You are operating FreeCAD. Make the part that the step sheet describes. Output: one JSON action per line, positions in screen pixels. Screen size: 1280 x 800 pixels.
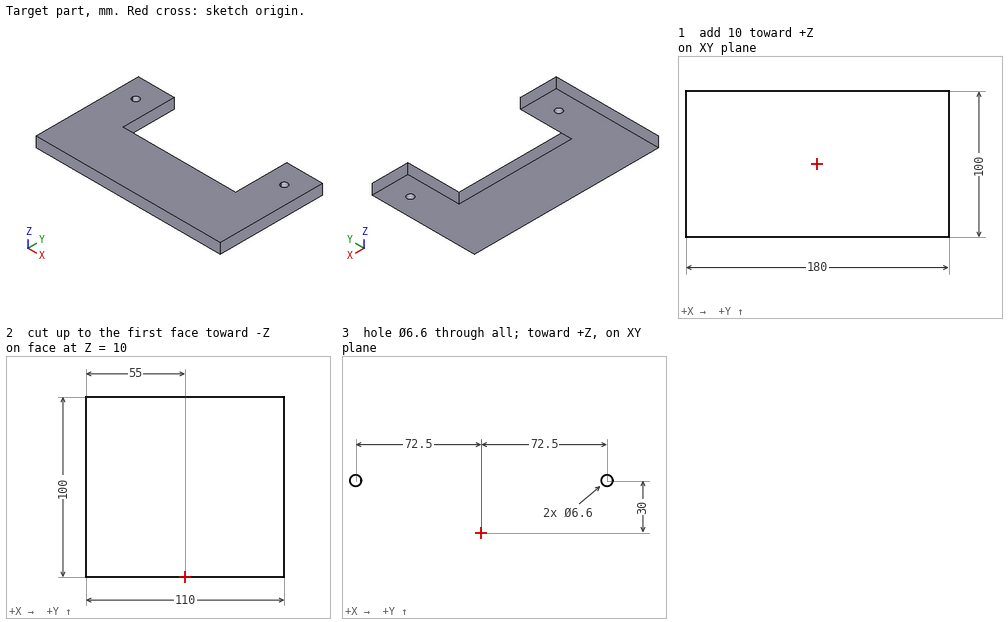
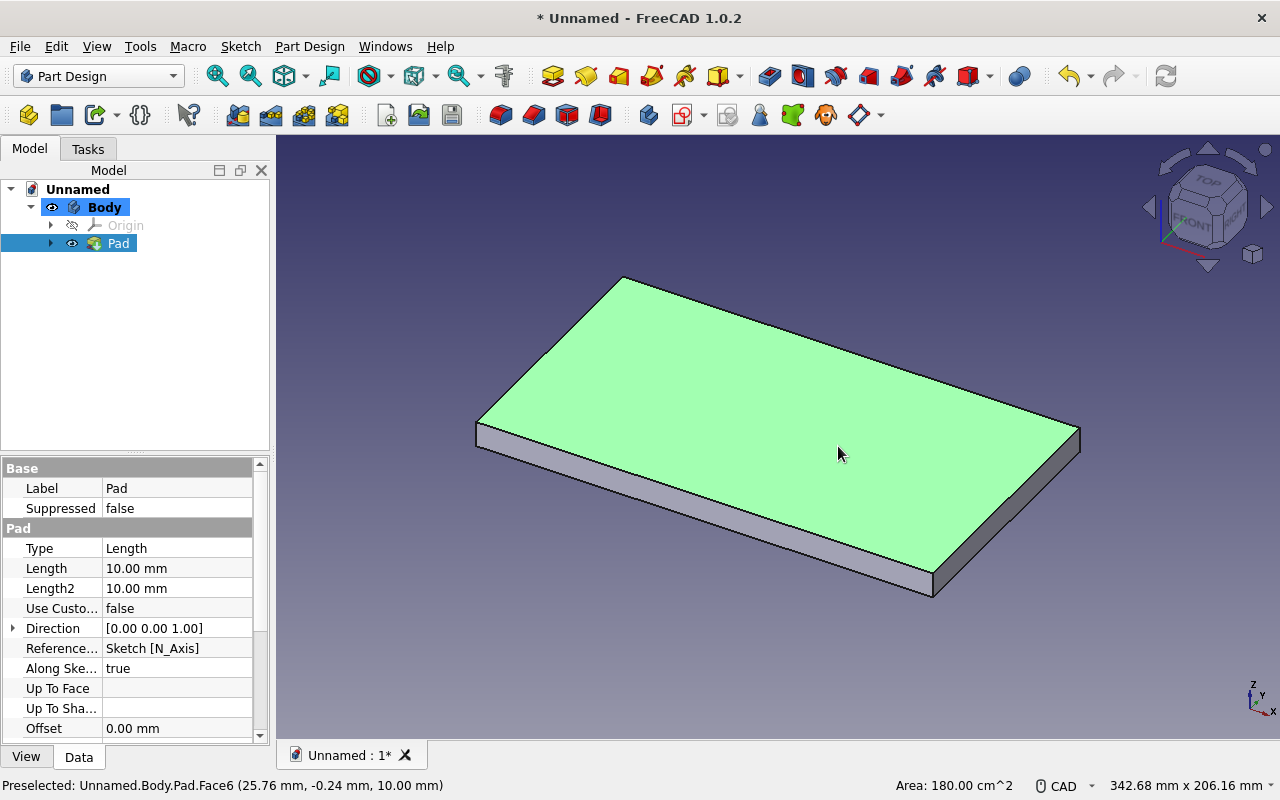
{"action": "left_click", "coordinate": [682, 116]}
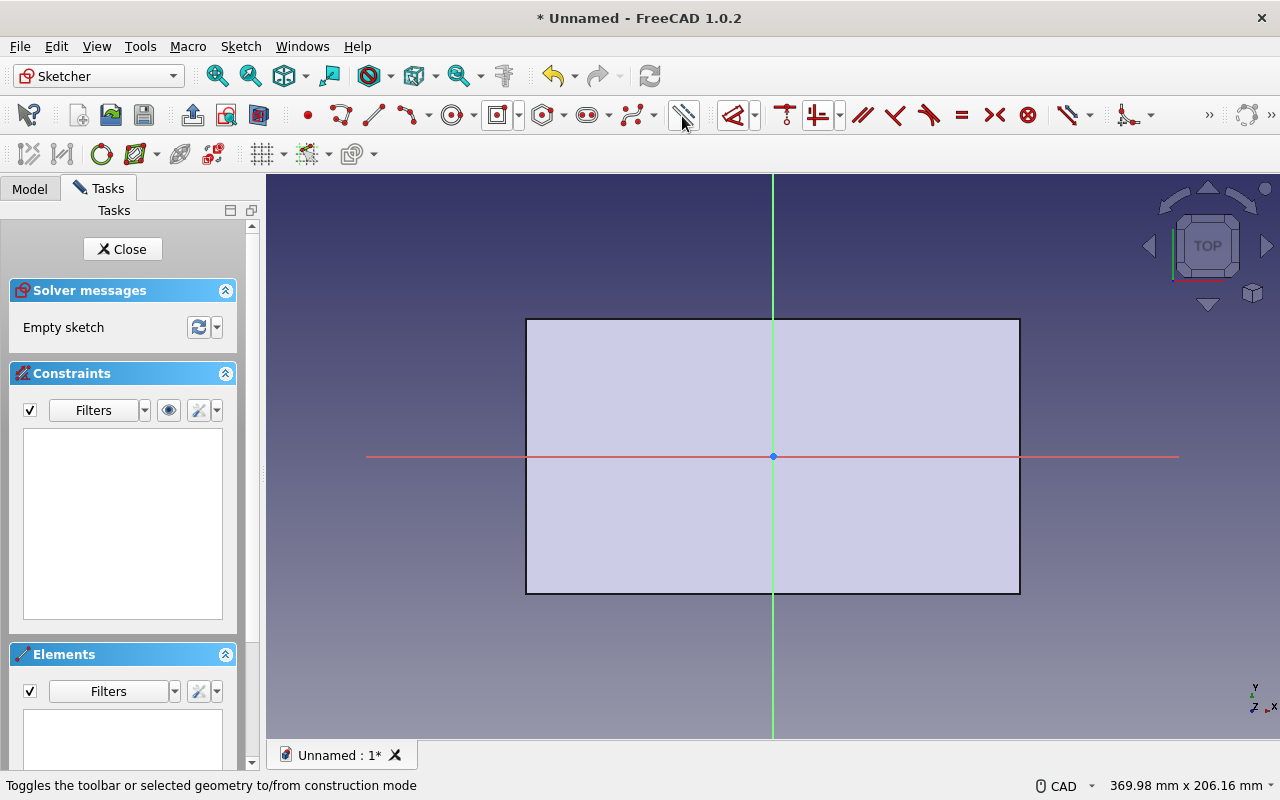
{"action": "scroll", "coordinate": [395, 711], "scroll_direction": "down", "scroll_amount": 1}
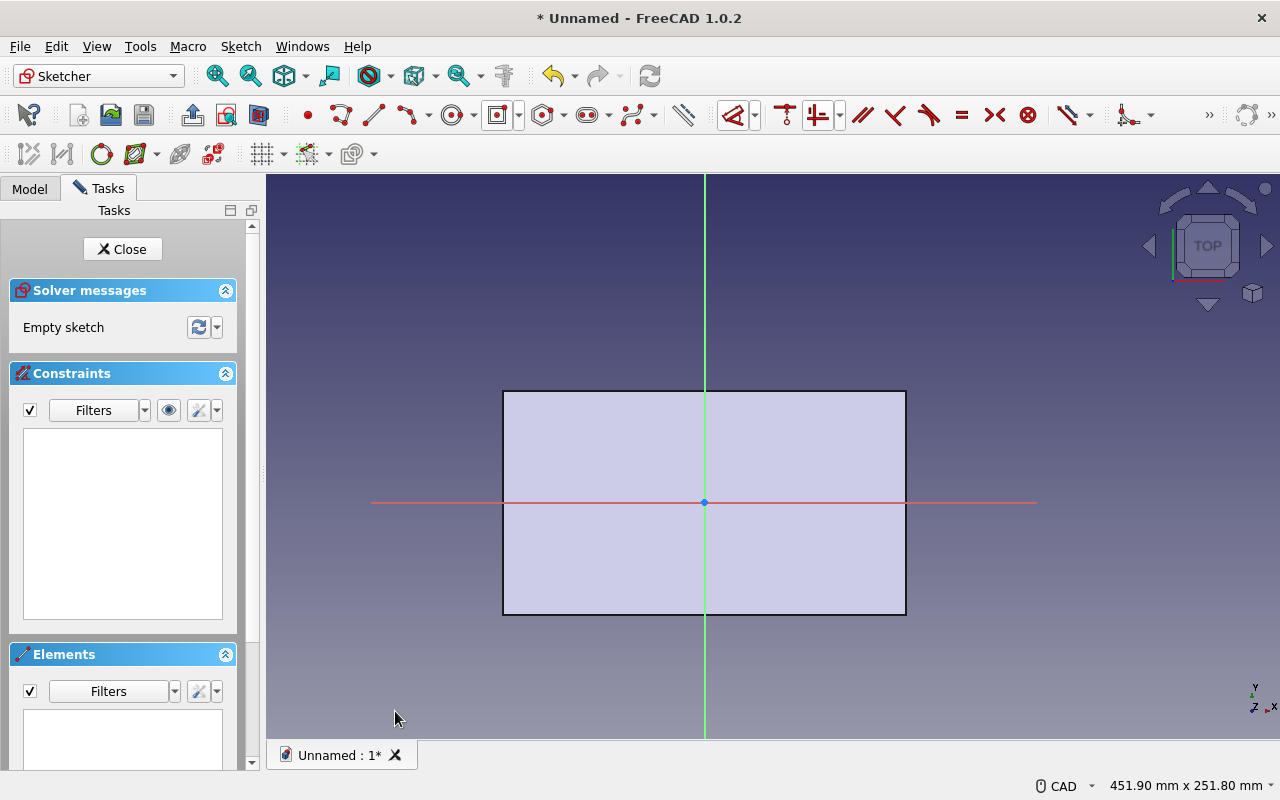
{"action": "scroll", "coordinate": [705, 257], "scroll_direction": "up", "scroll_amount": 2}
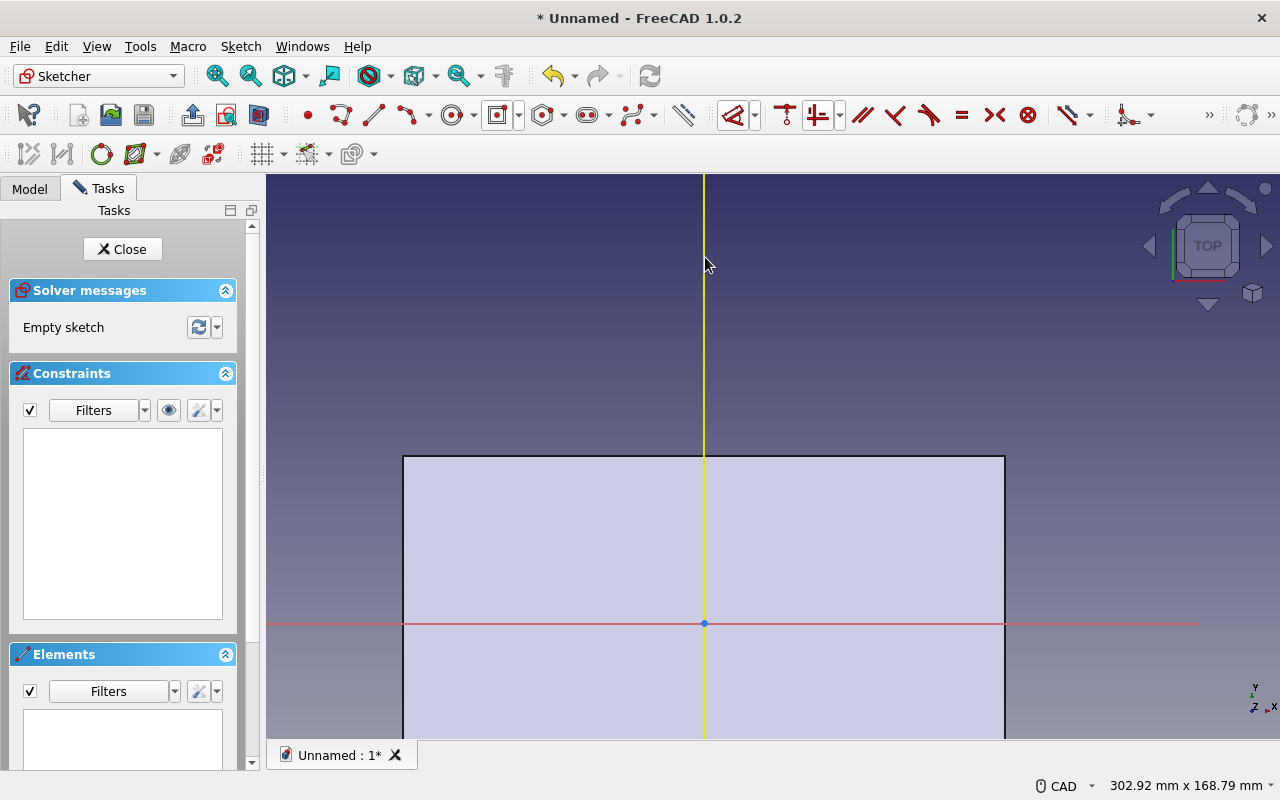
{"action": "key", "text": "g r"}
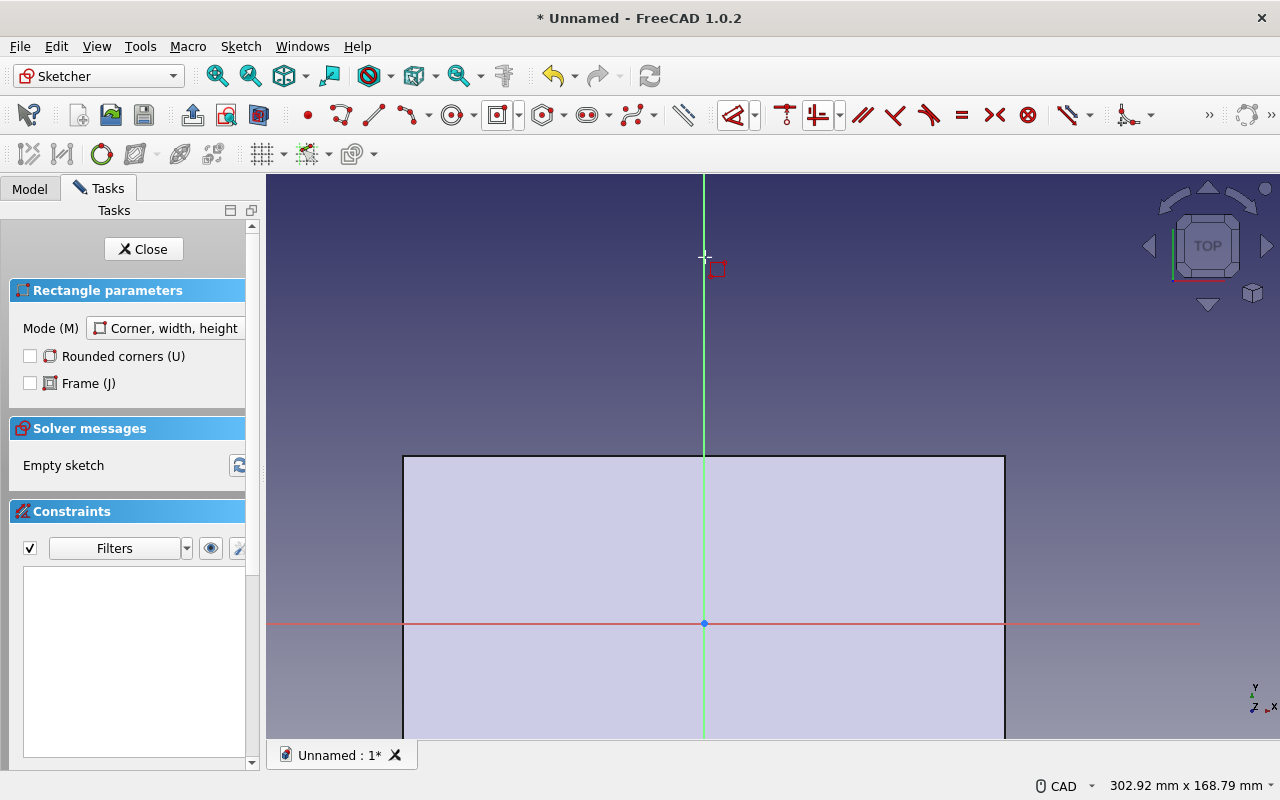
{"action": "left_click", "coordinate": [520, 289]}
{"action": "left_click", "coordinate": [888, 624]}
{"action": "key", "text": "Escape"}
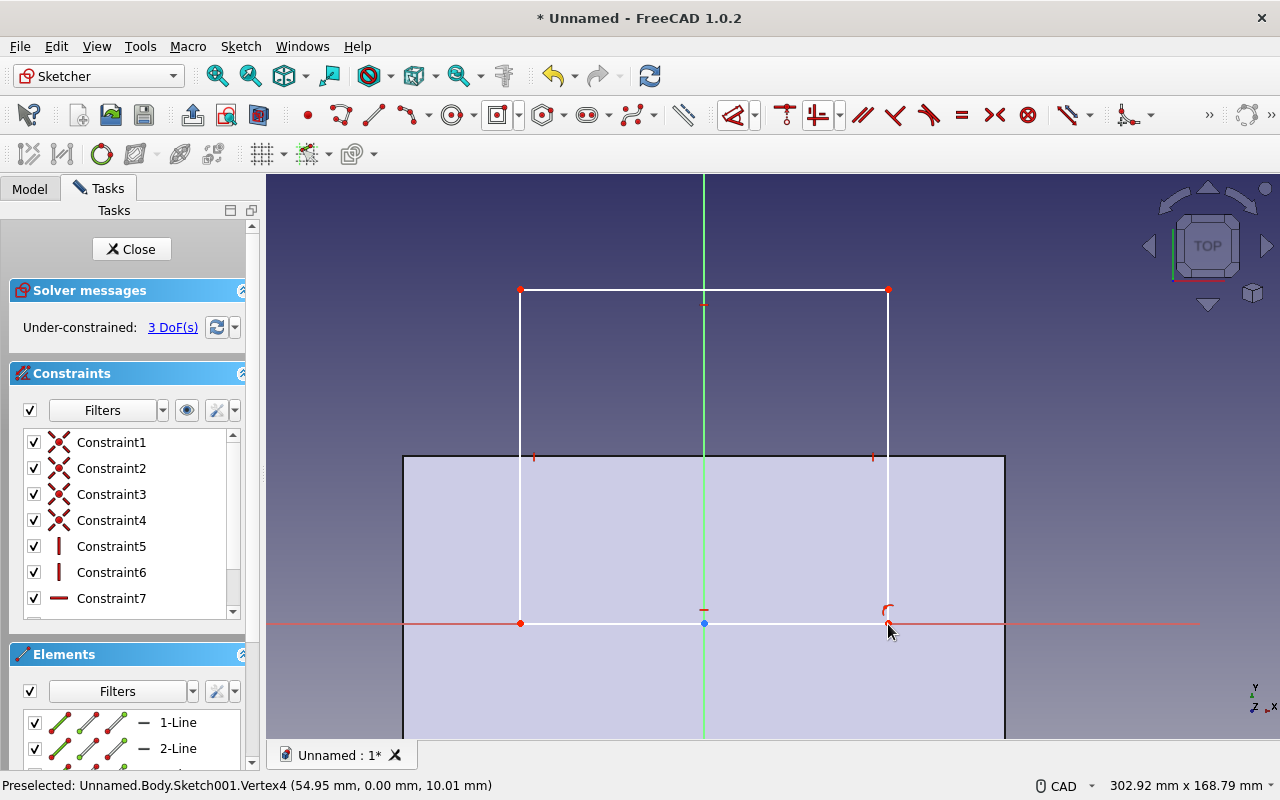
{"action": "left_click", "coordinate": [520, 390]}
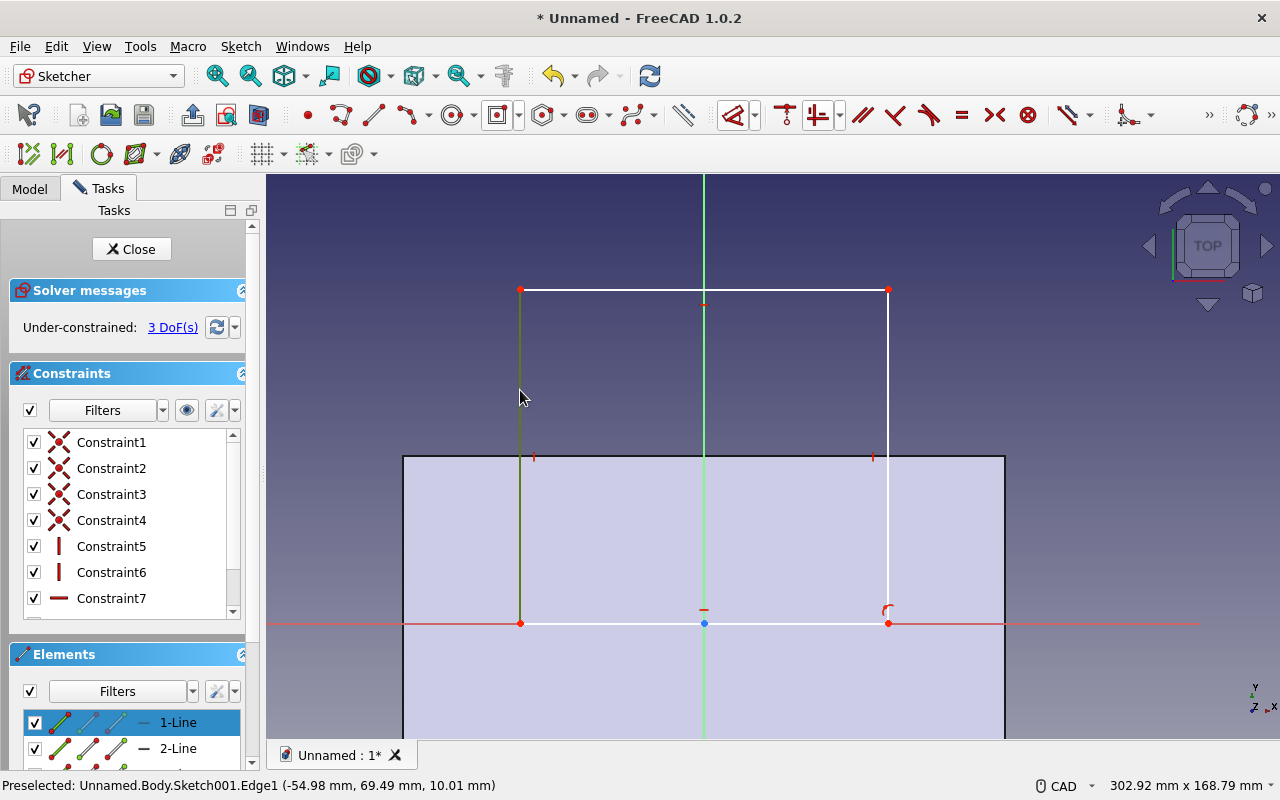
{"action": "key", "text": "i"}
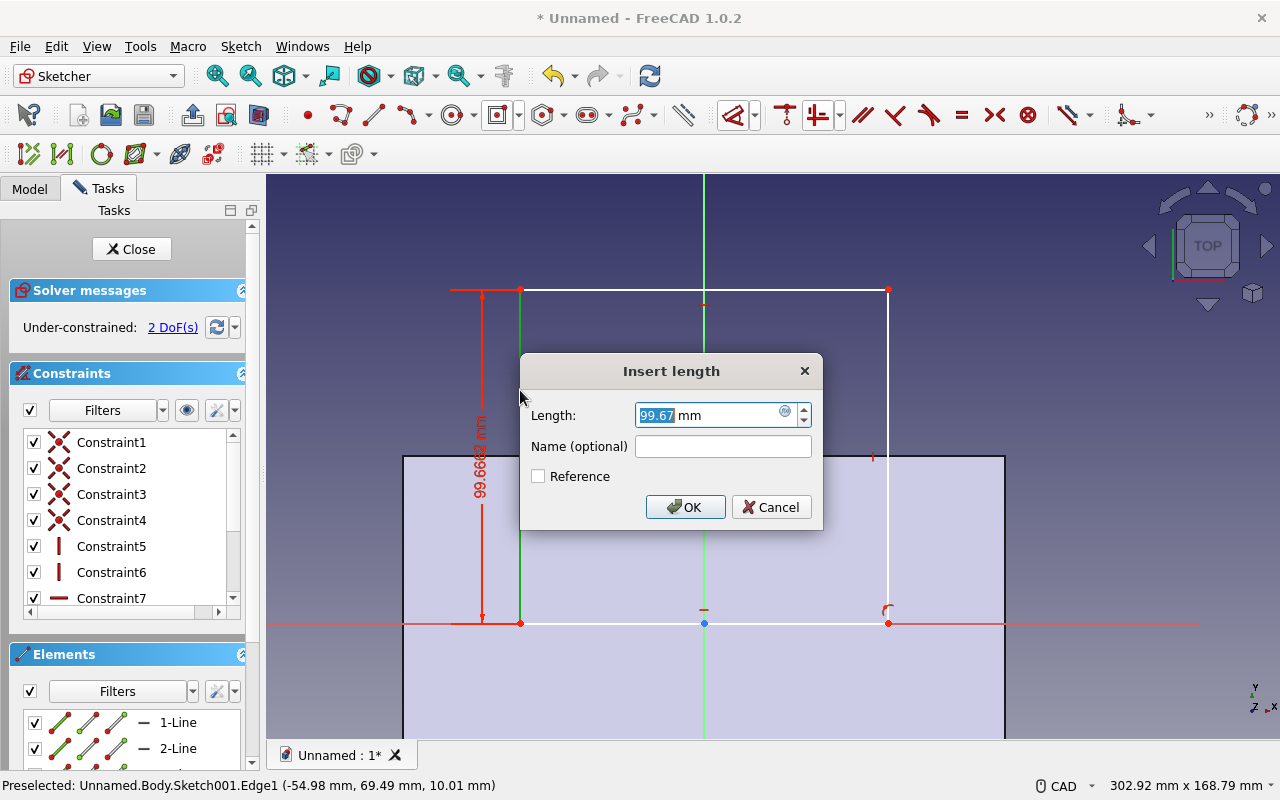
{"action": "type", "text": "100"}
{"action": "key", "text": "Return"}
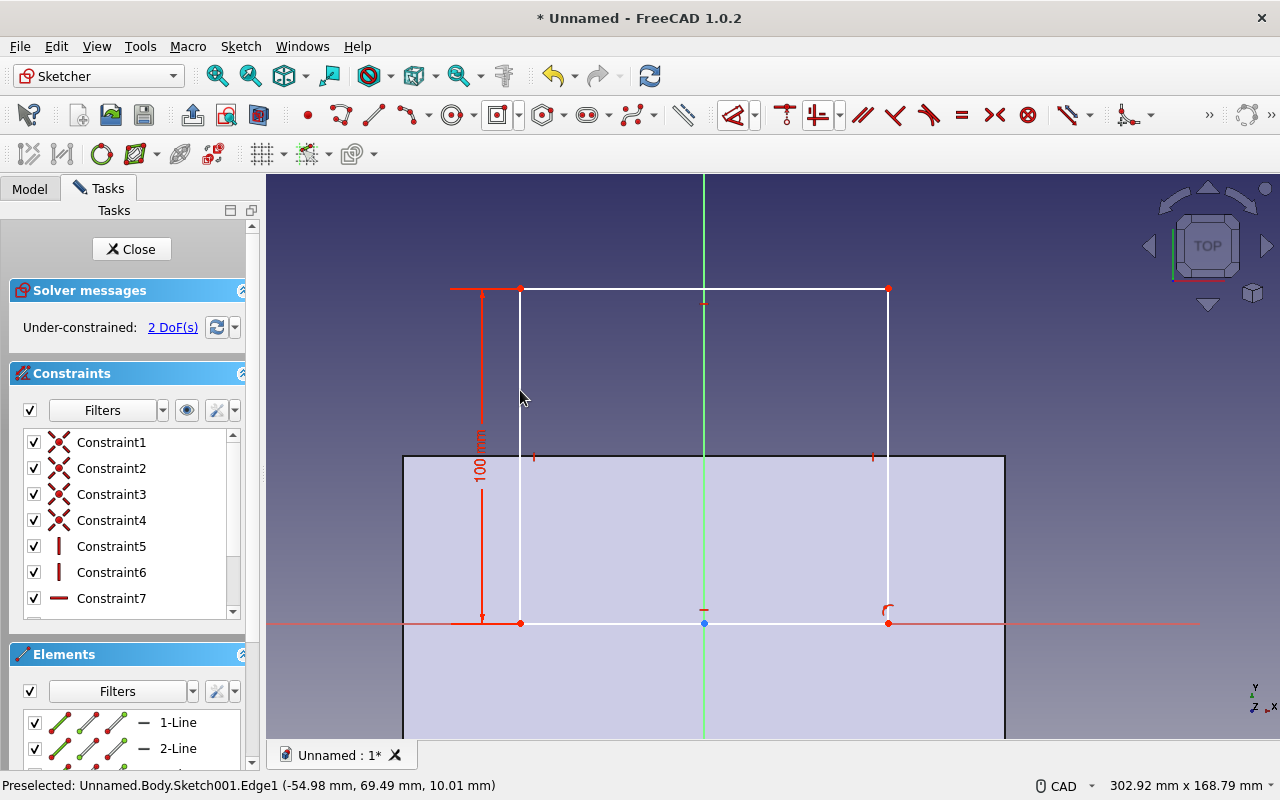
{"action": "left_click", "coordinate": [630, 624]}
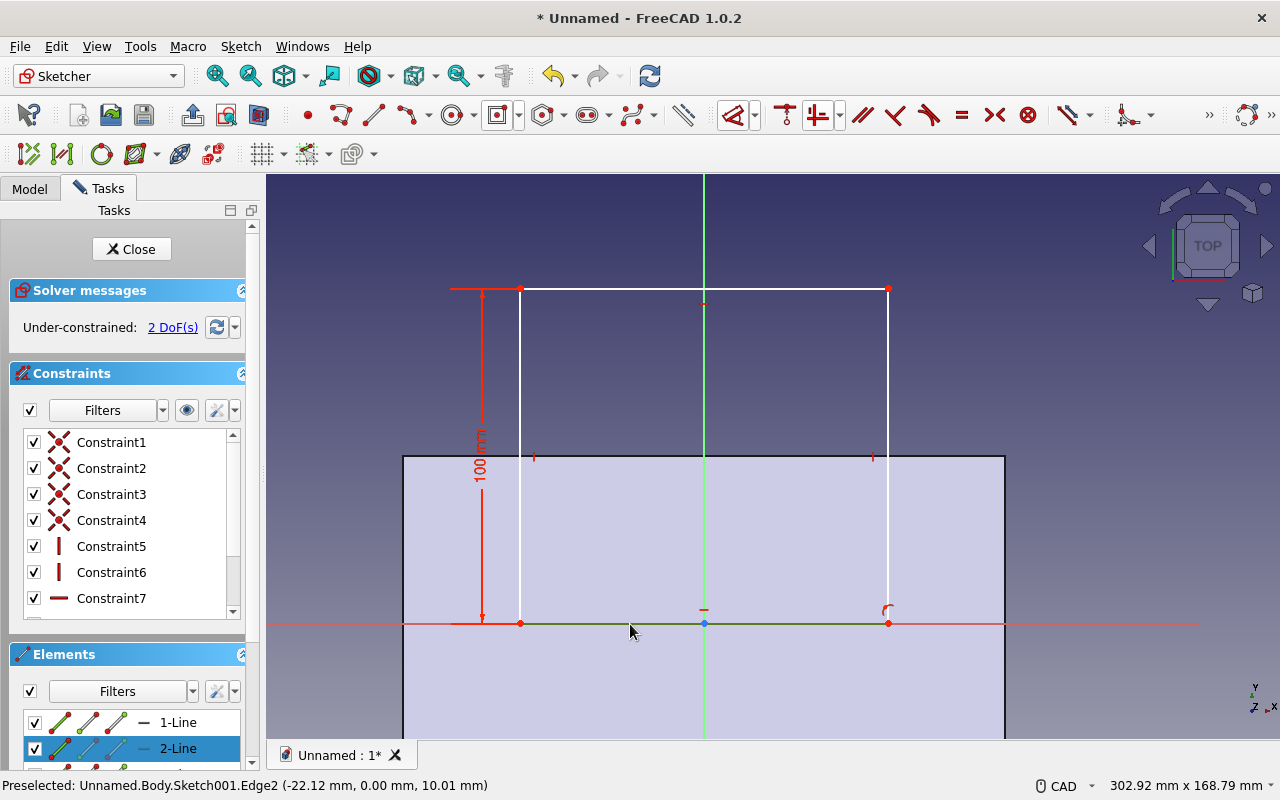
{"action": "key", "text": "l"}